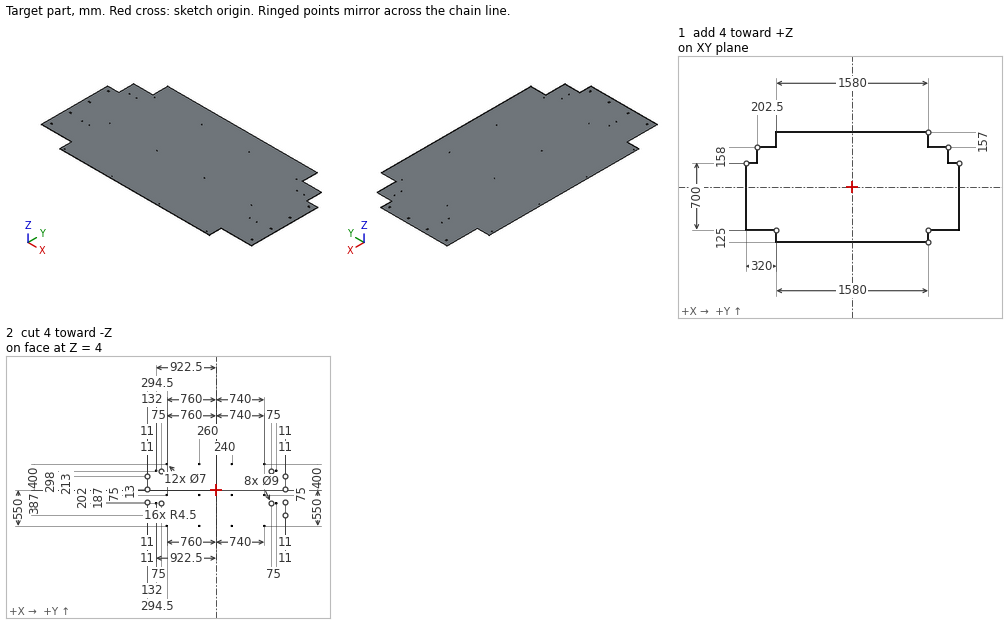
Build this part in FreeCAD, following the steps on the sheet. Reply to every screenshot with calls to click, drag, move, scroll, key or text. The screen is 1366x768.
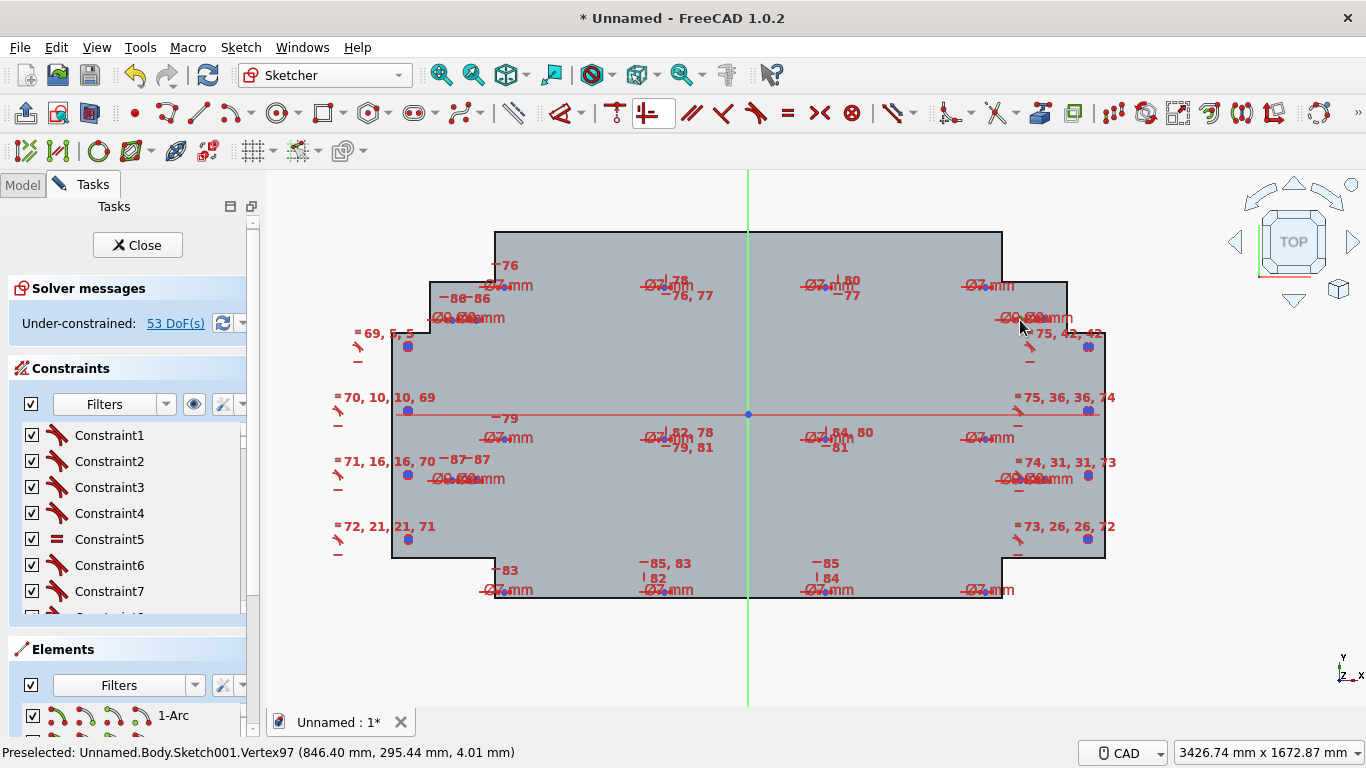
click(1044, 320)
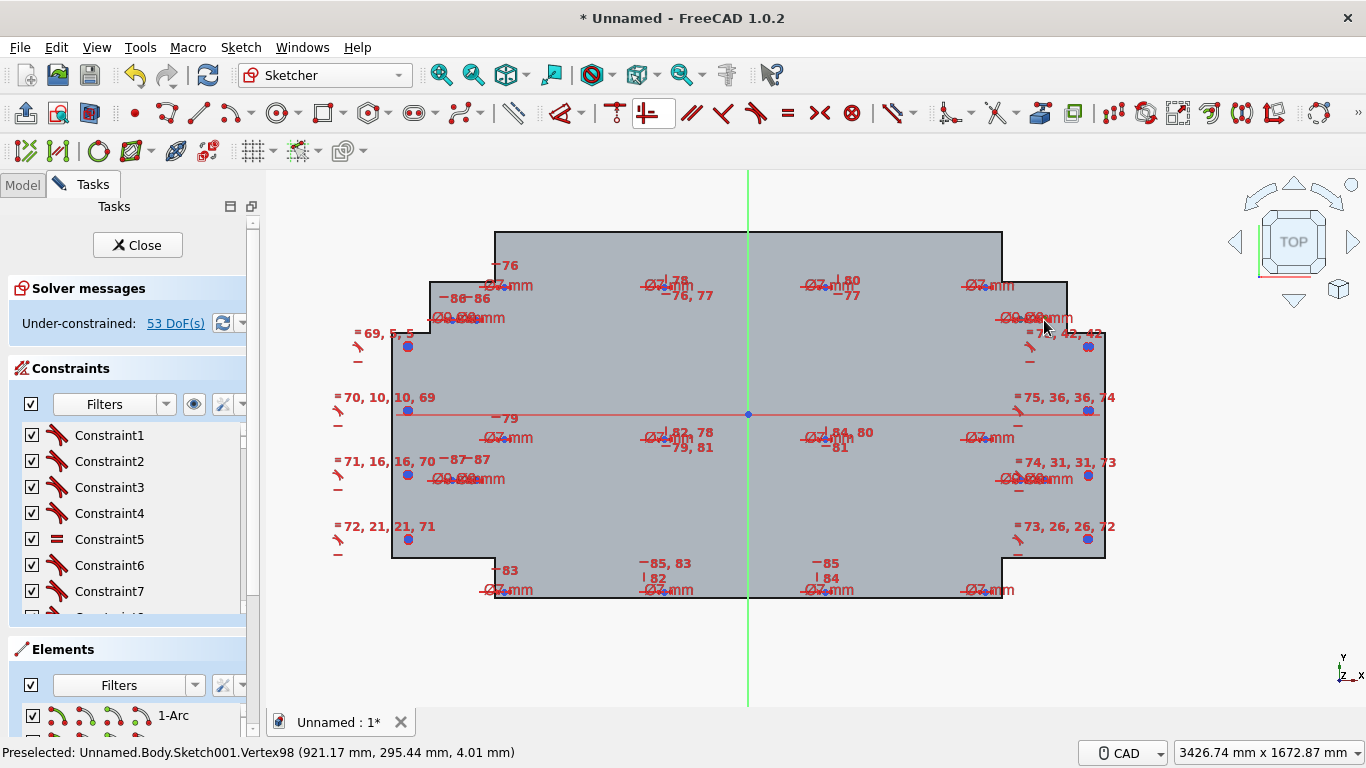
key(h)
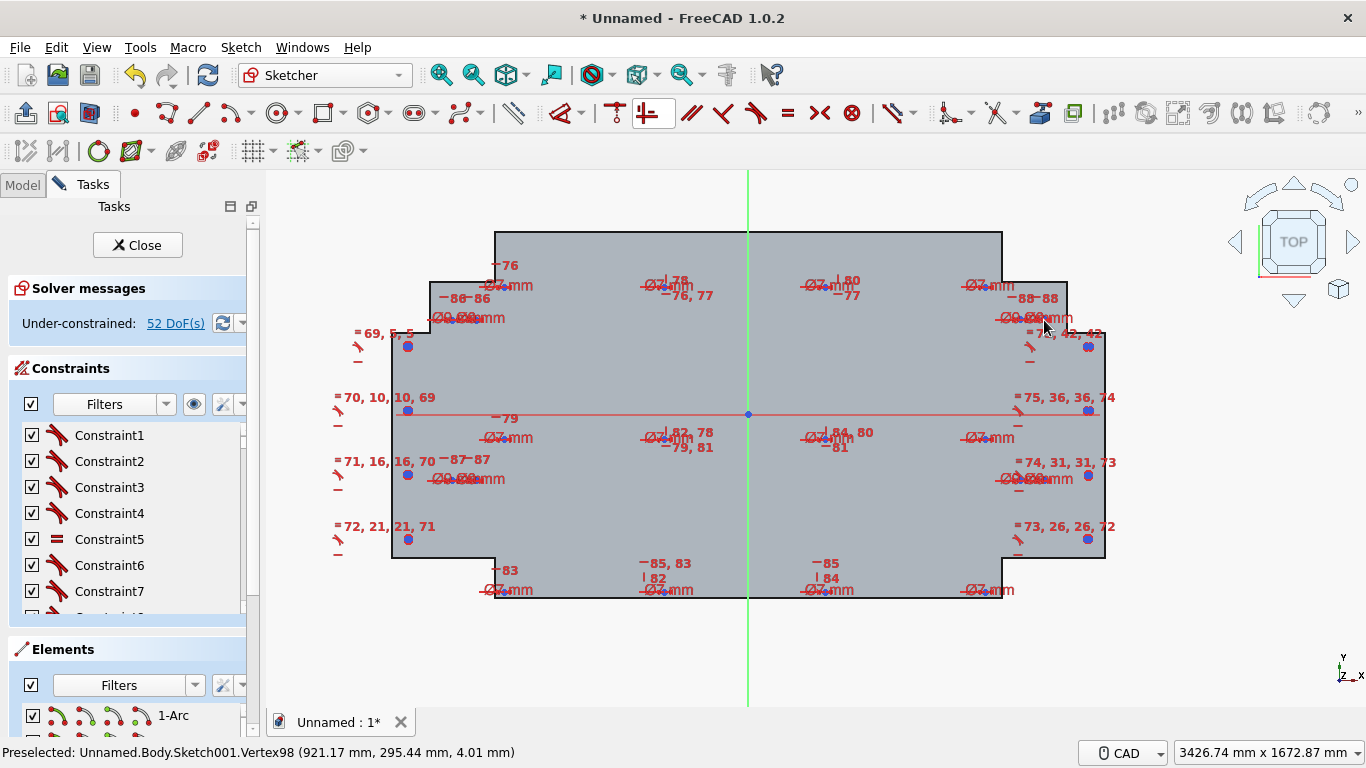
click(1020, 481)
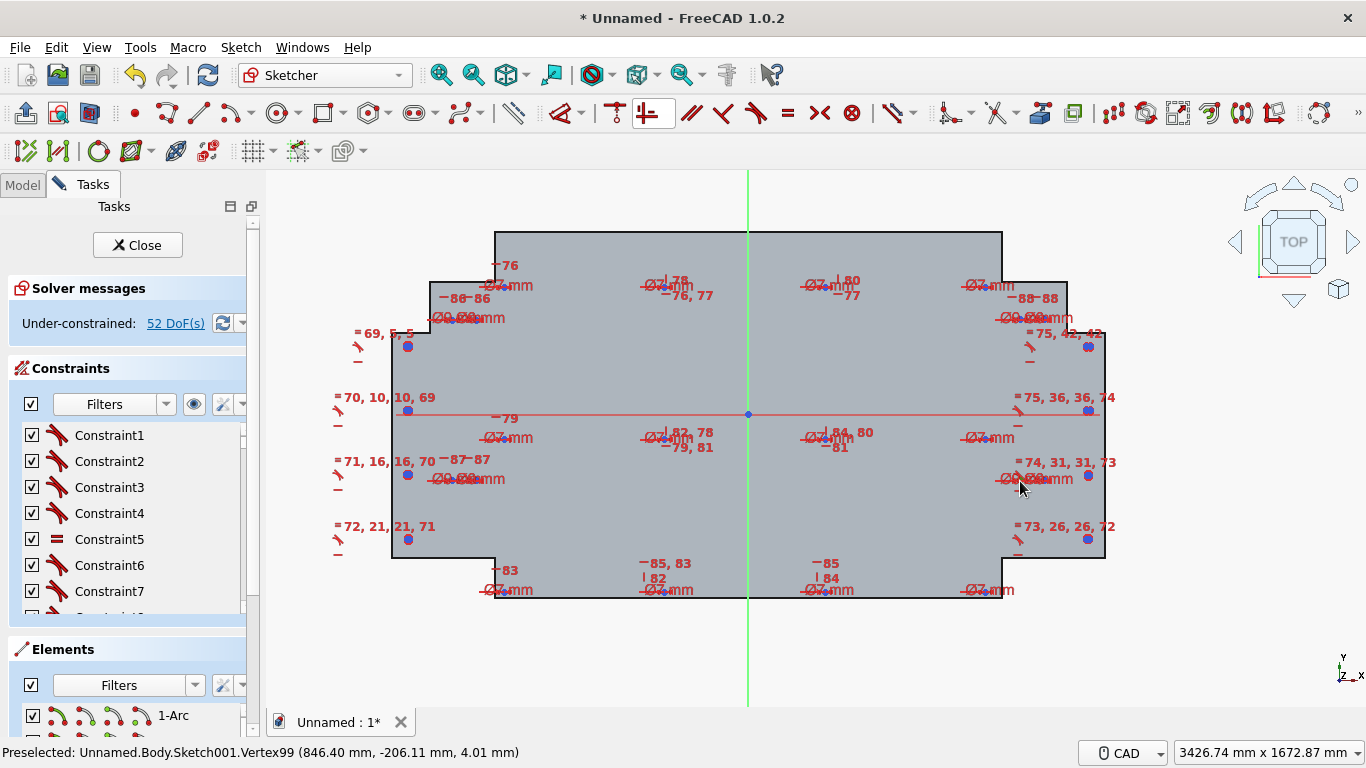
click(1044, 481)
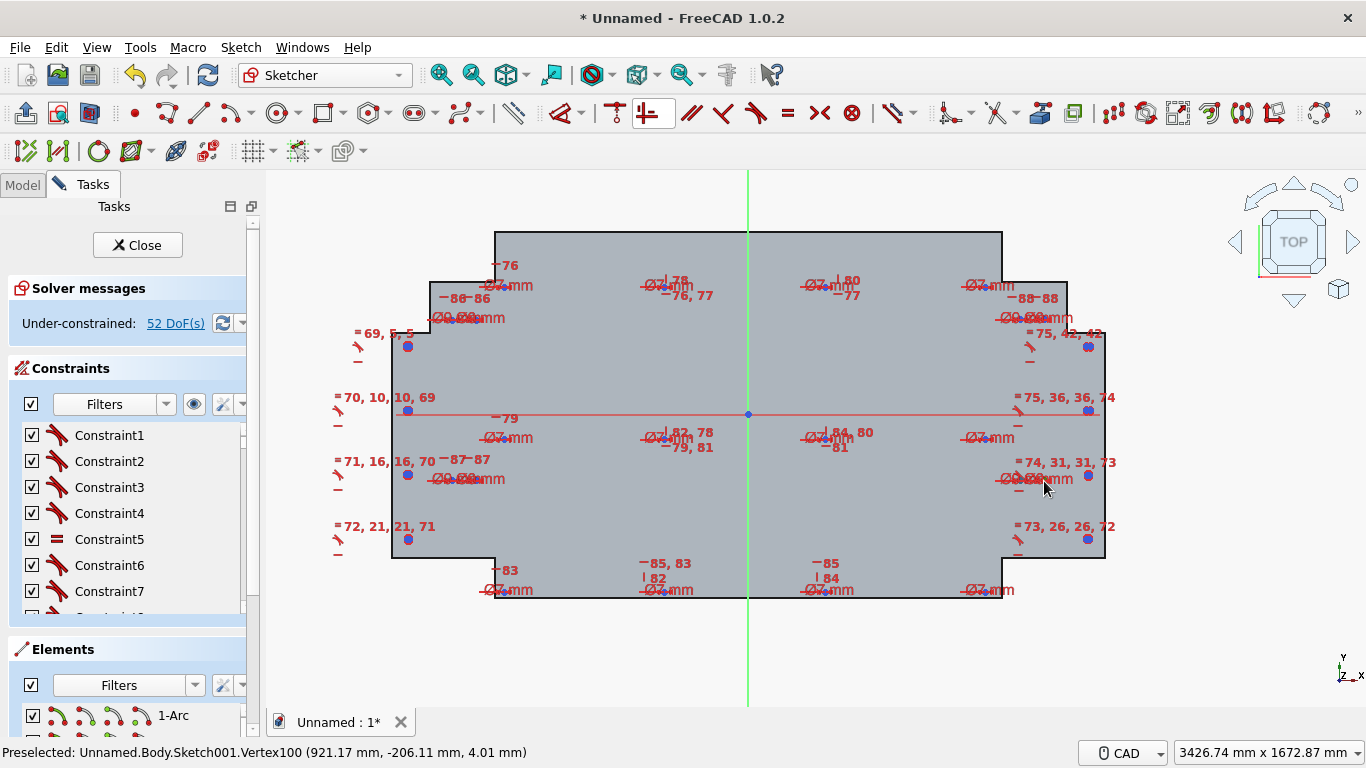
click(670, 114)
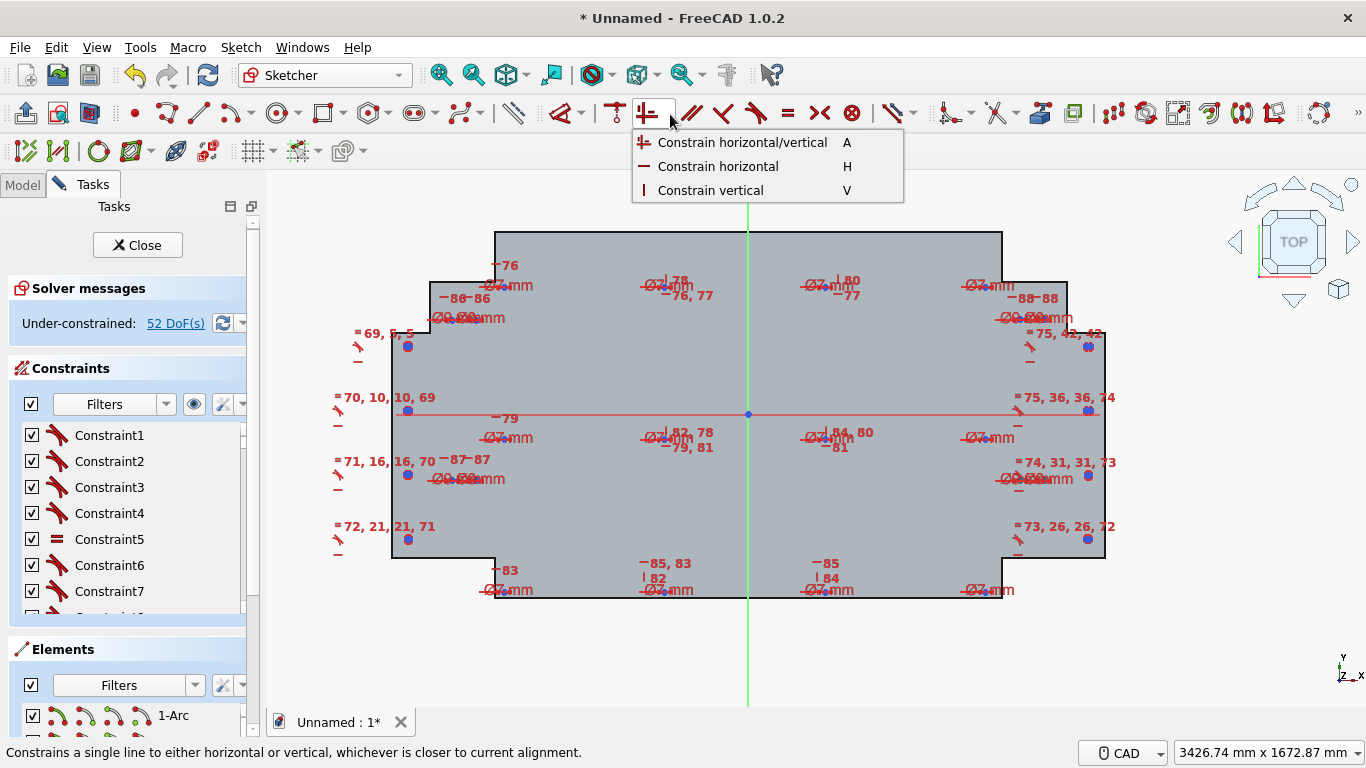
click(768, 166)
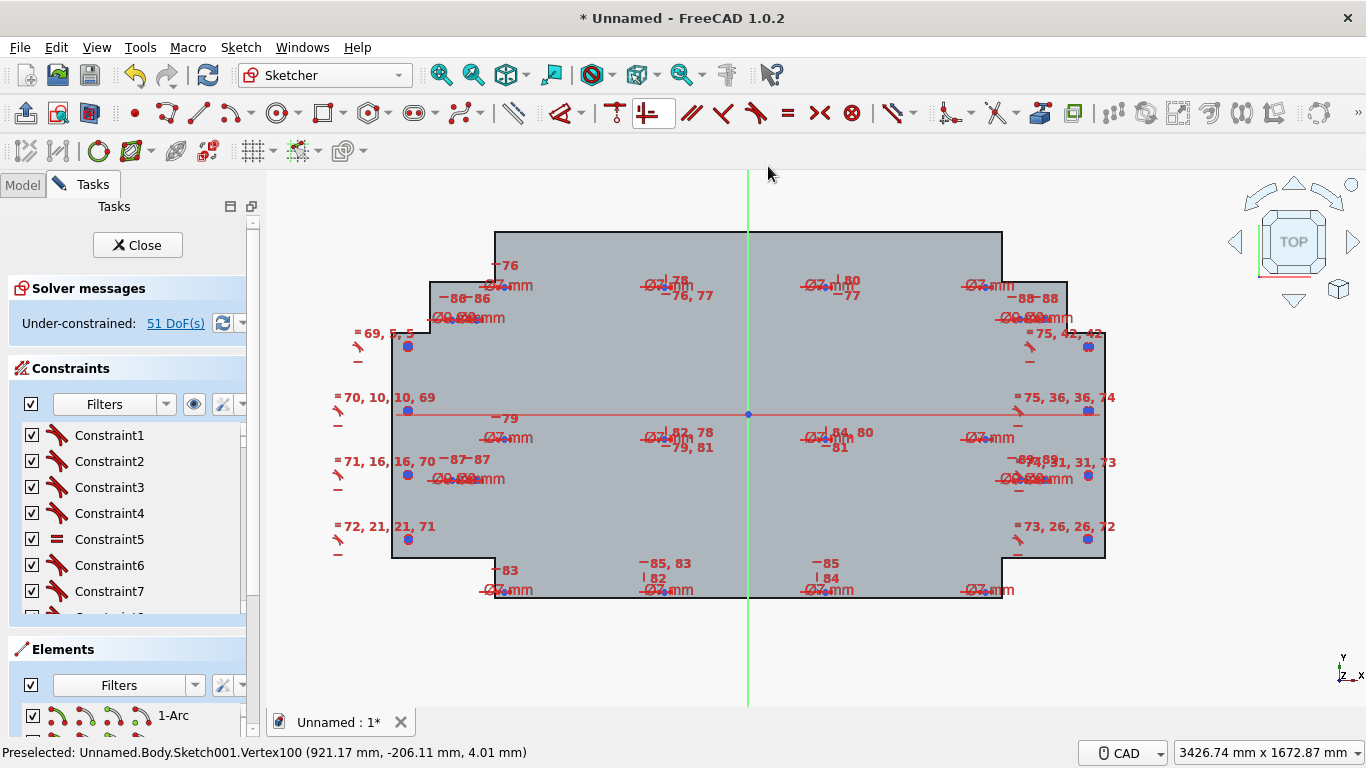
scroll(409, 539, up, 11)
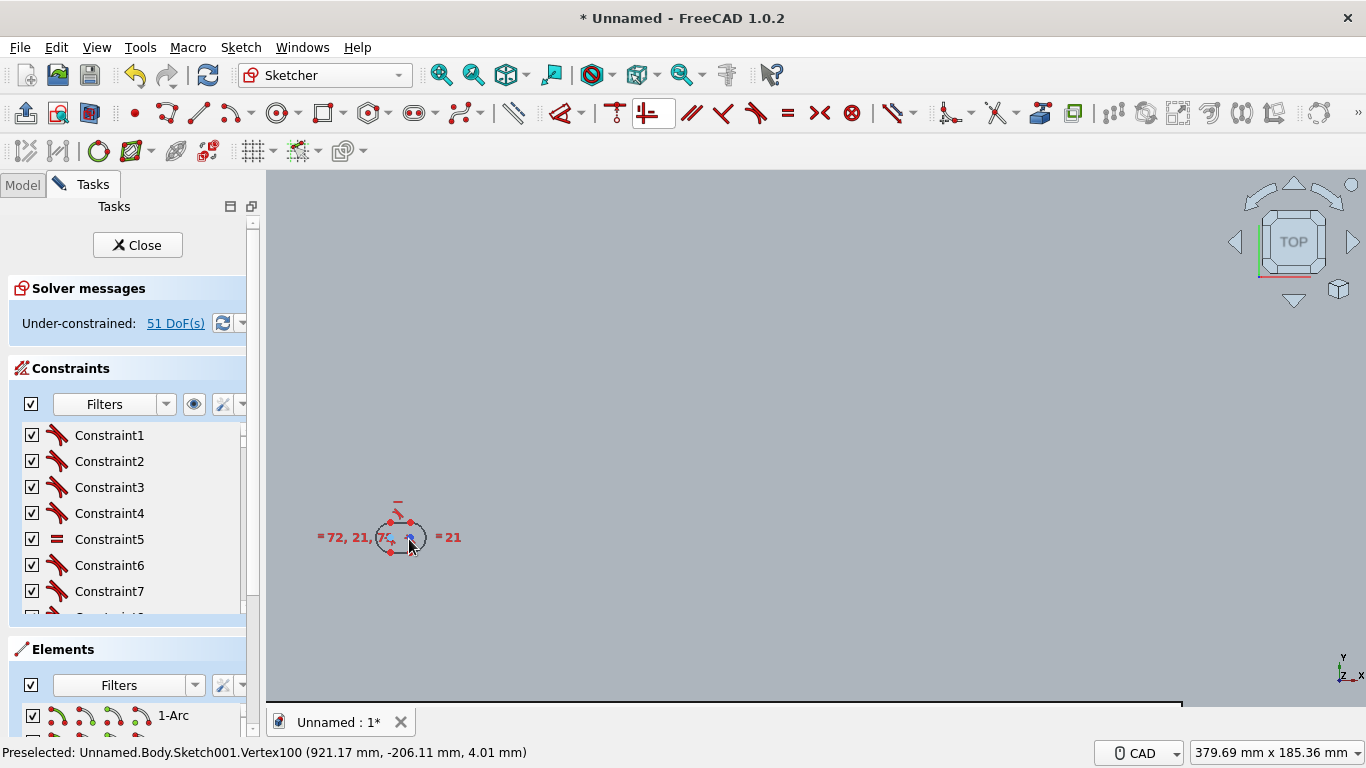
click(411, 538)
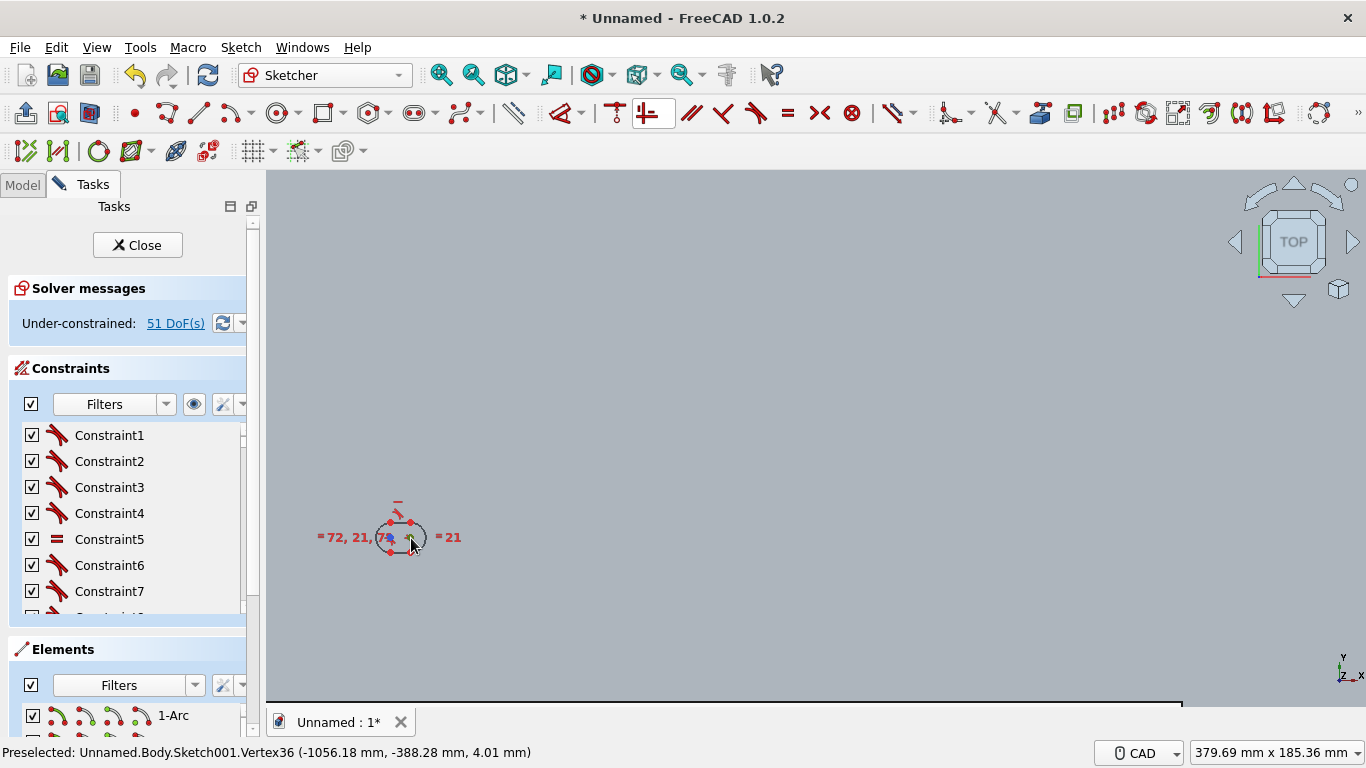
scroll(408, 539, down, 11)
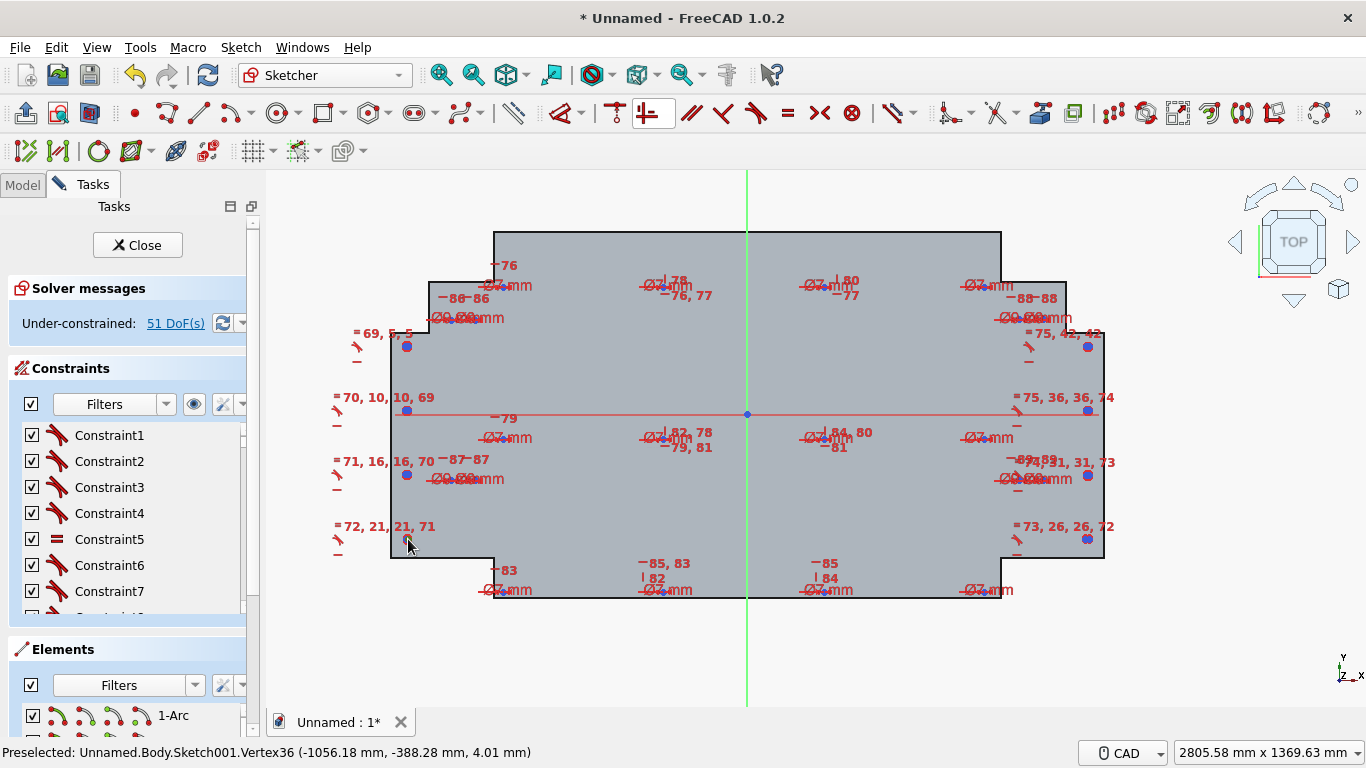
scroll(1086, 539, up, 11)